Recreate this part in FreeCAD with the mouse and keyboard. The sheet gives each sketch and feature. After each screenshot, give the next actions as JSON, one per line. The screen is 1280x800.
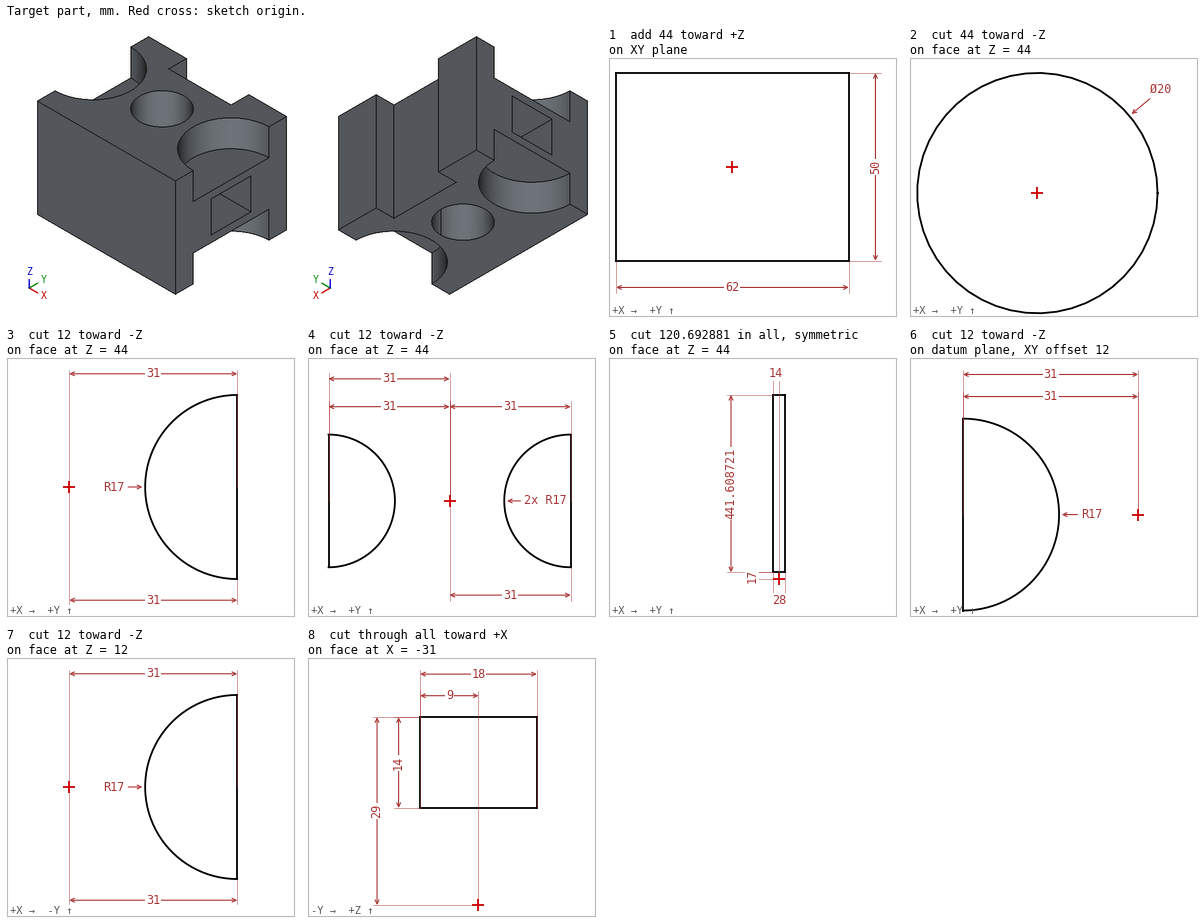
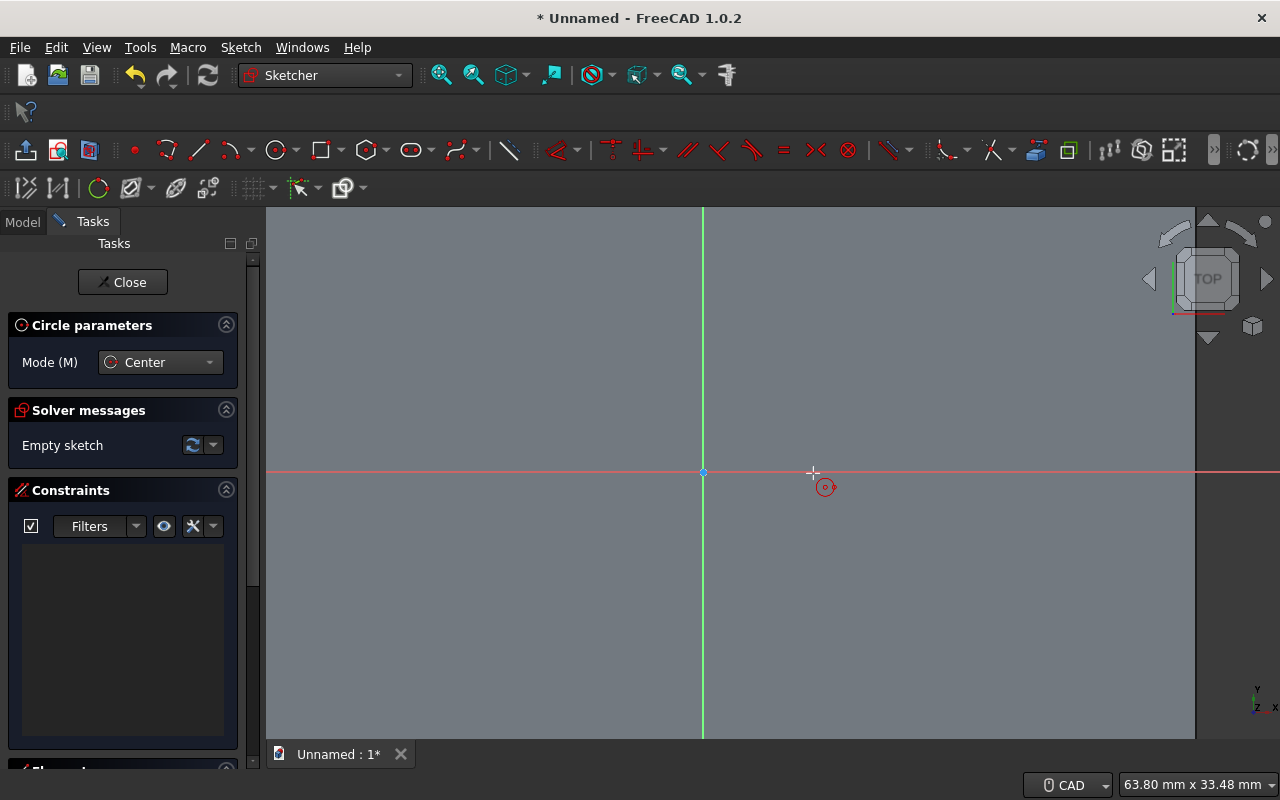
{"action": "left_click", "coordinate": [703, 472]}
{"action": "left_click", "coordinate": [816, 360]}
{"action": "key", "text": "Escape"}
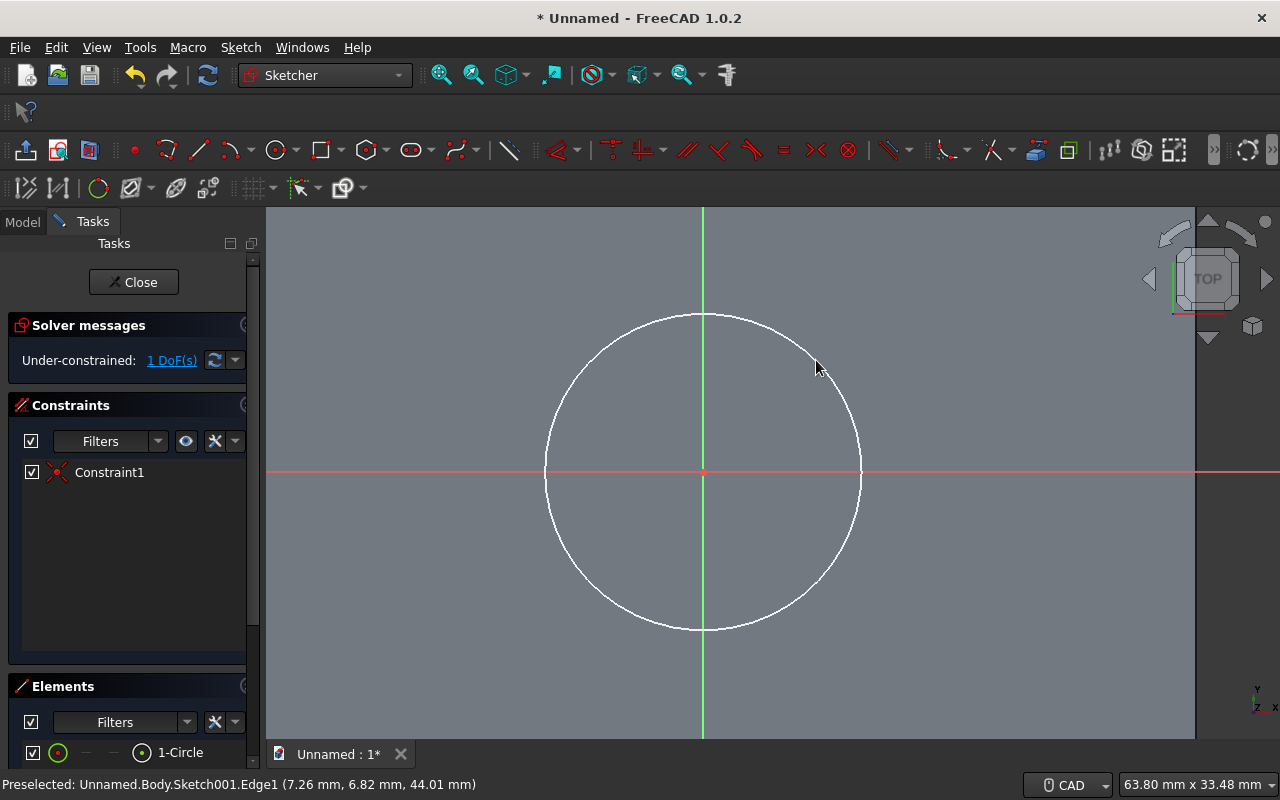
{"action": "key", "text": "d"}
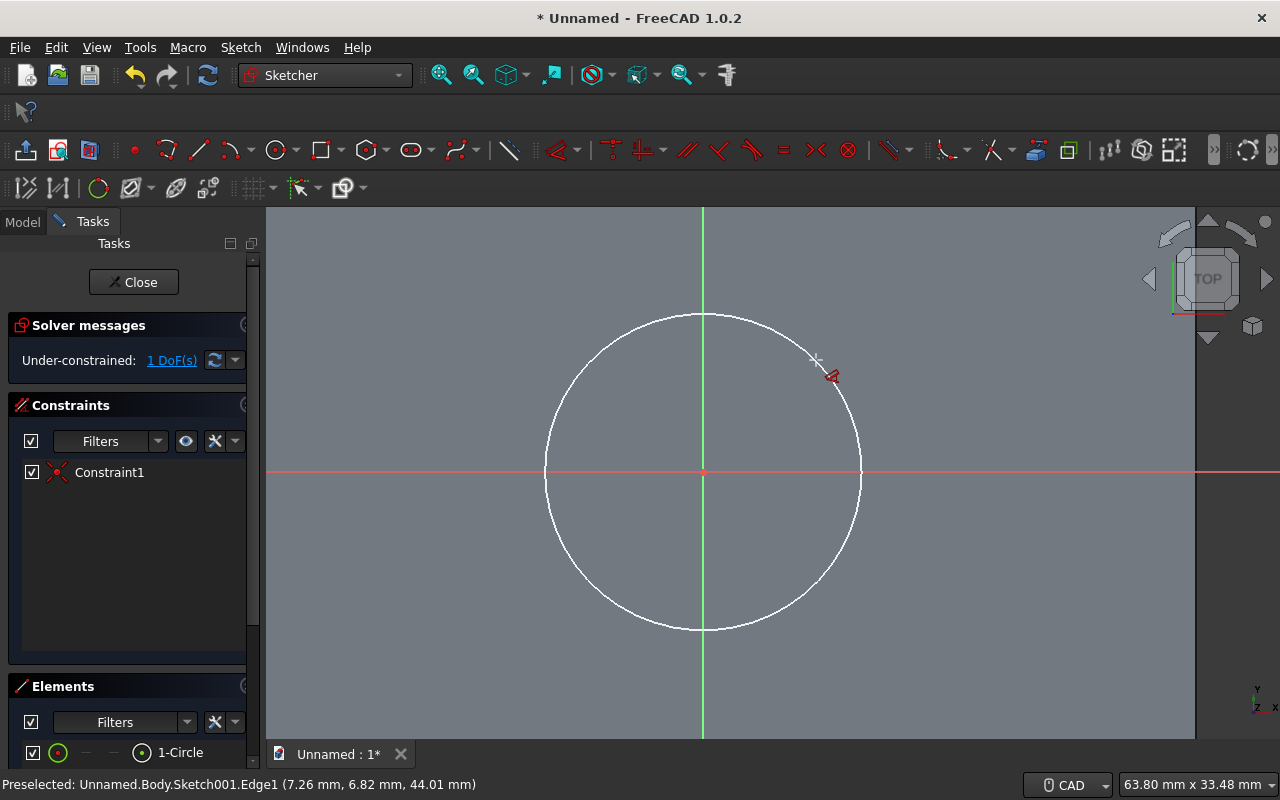
{"action": "left_click", "coordinate": [815, 360]}
{"action": "left_click", "coordinate": [838, 337]}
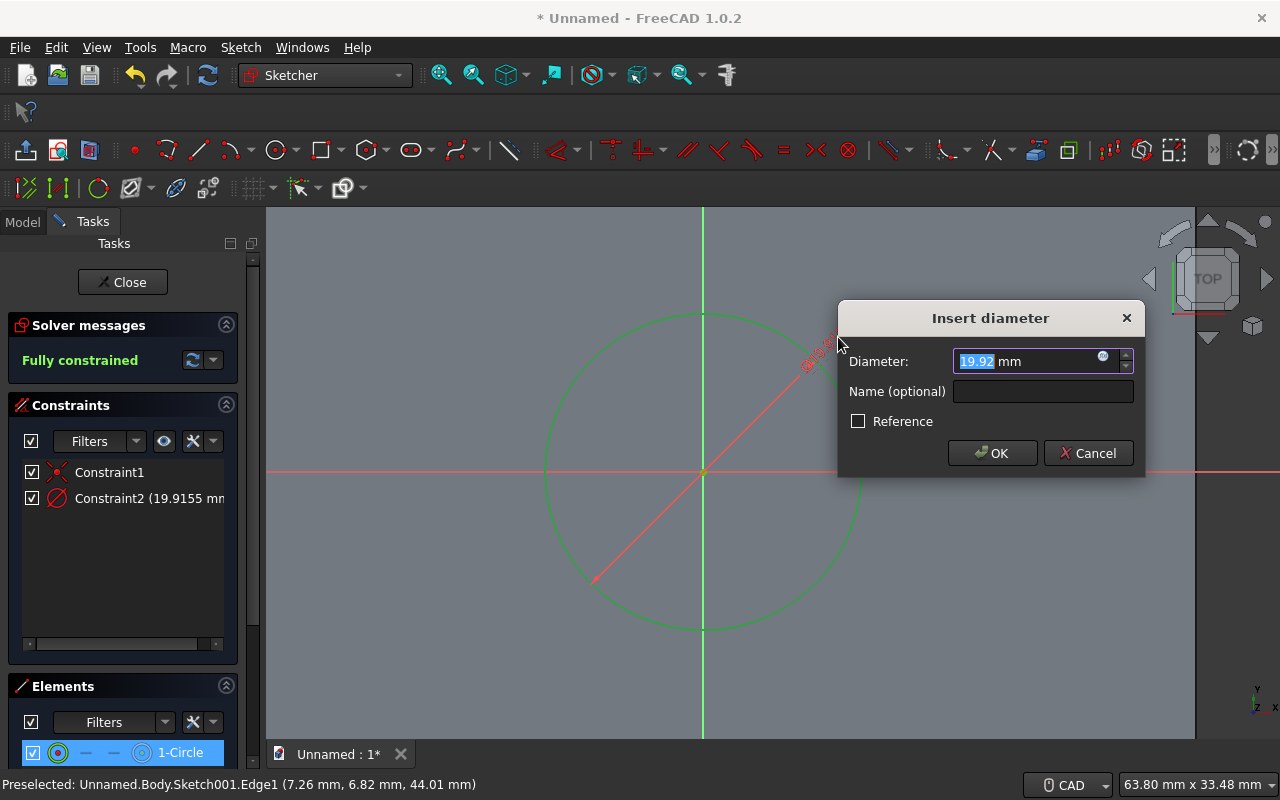
{"action": "type", "text": "20"}
{"action": "key", "text": "Return"}
{"action": "key", "text": "Escape"}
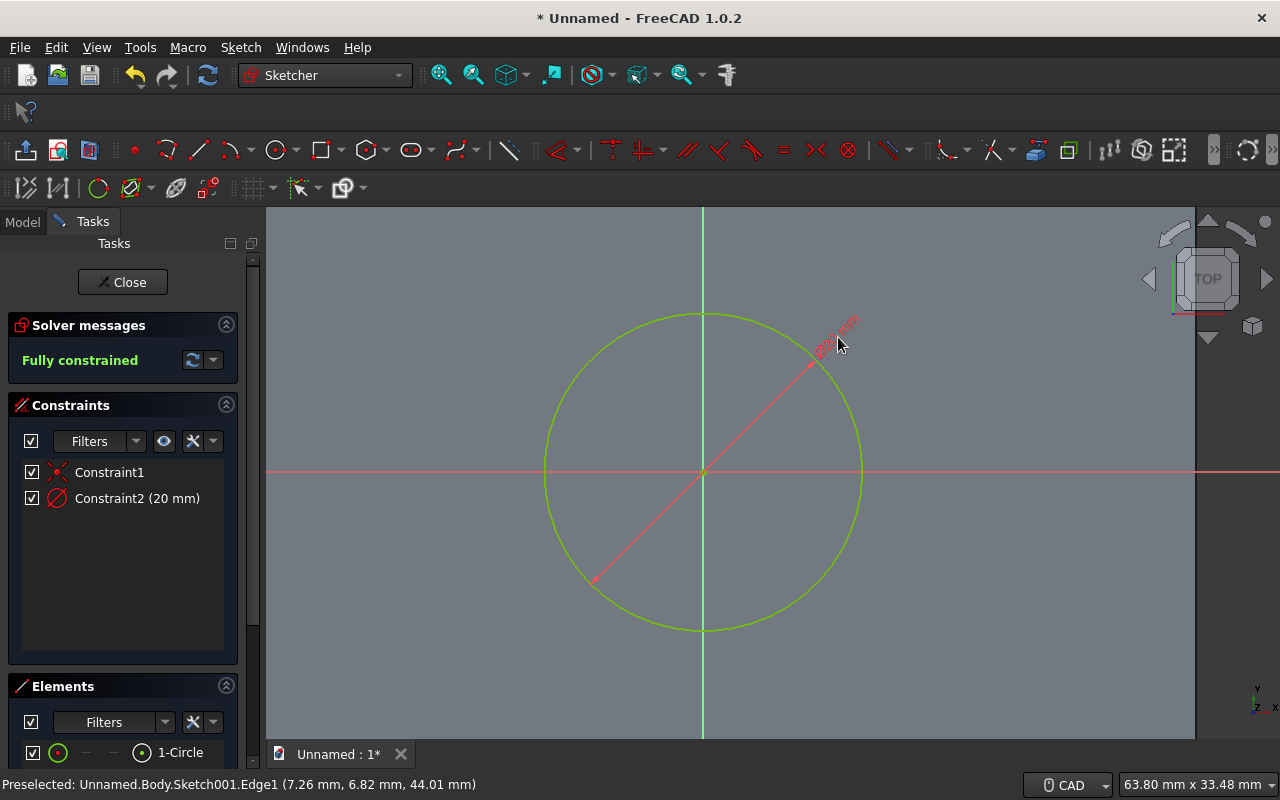
{"action": "left_click", "coordinate": [123, 282]}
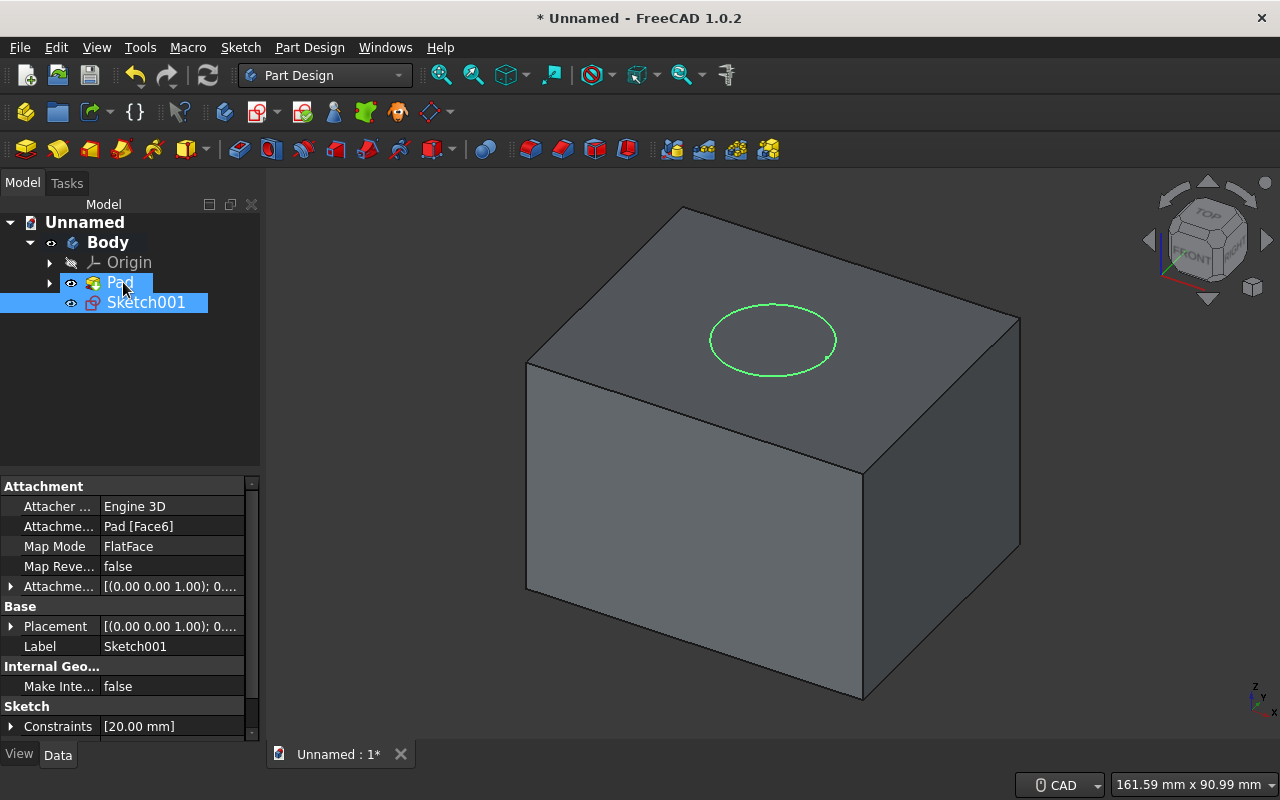
{"action": "left_click", "coordinate": [240, 150]}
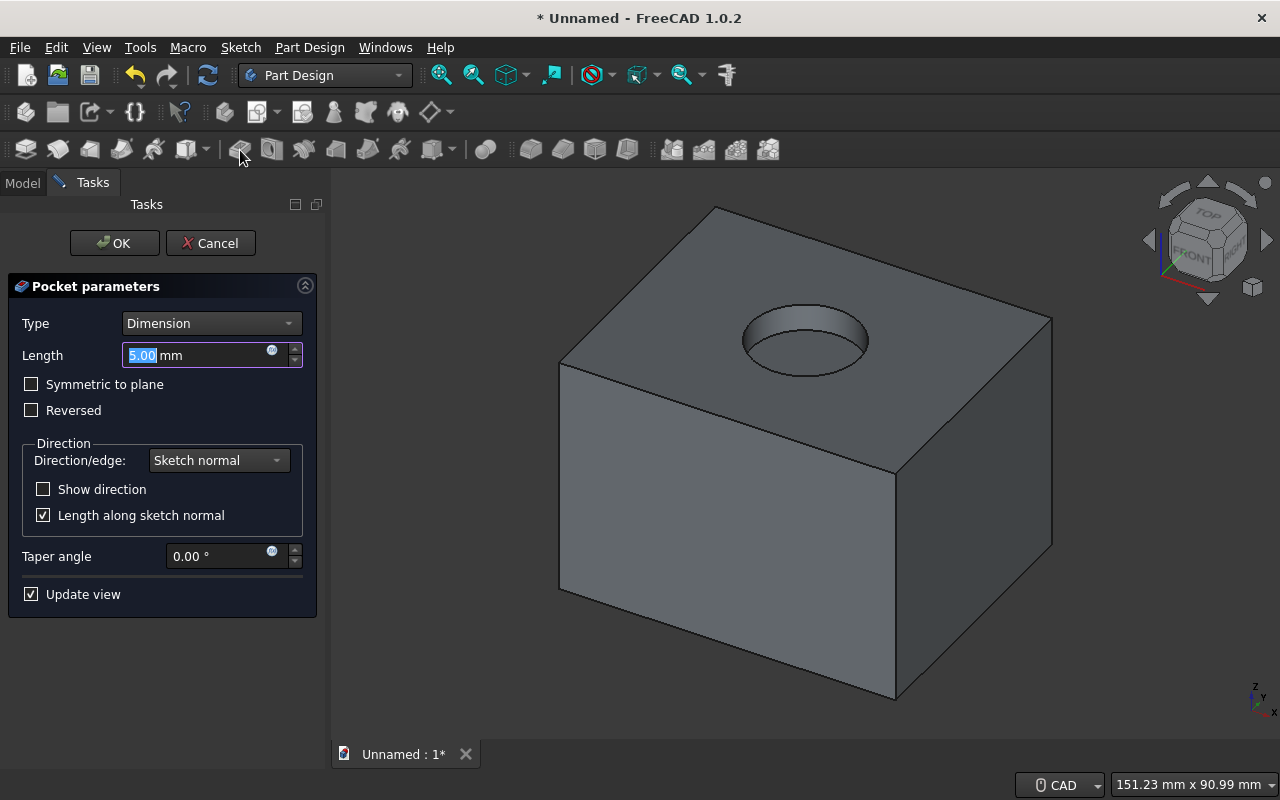
{"action": "type", "text": "44"}
{"action": "key", "text": "Tab"}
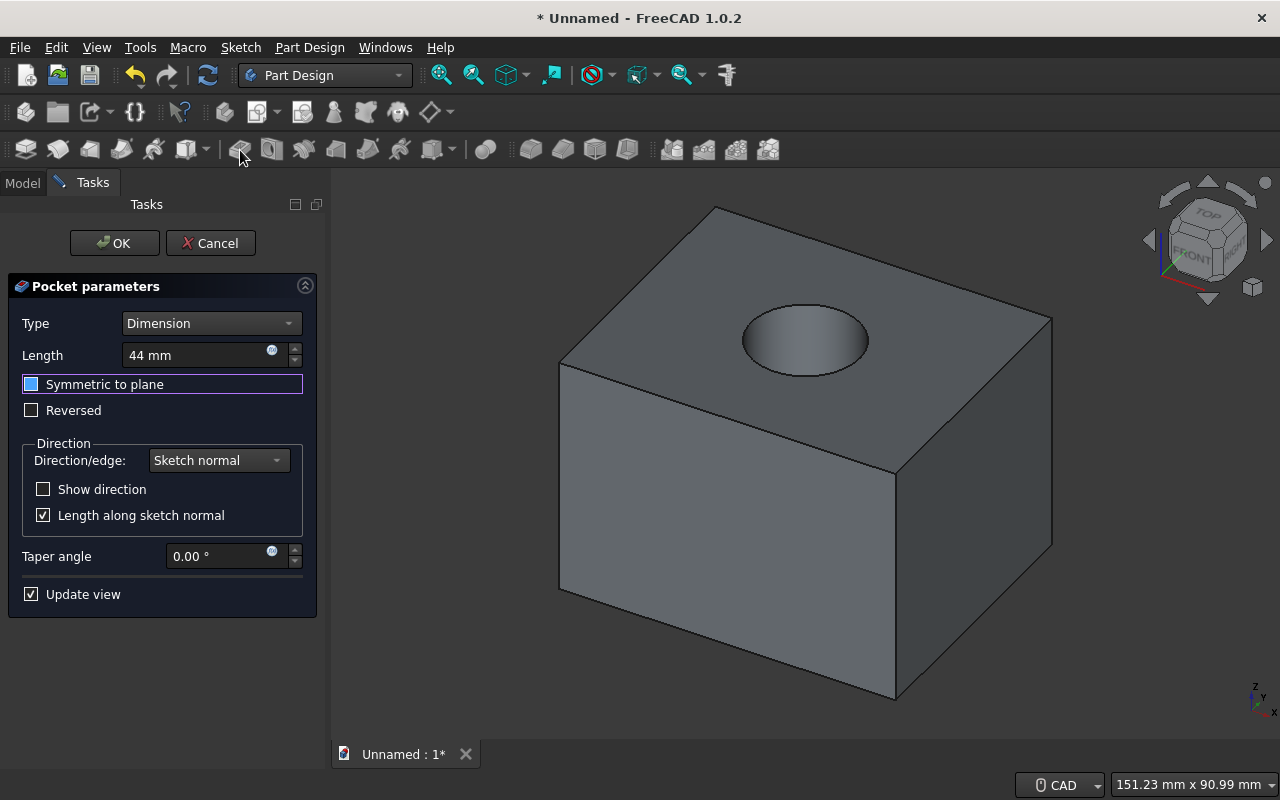
{"action": "left_click", "coordinate": [115, 243]}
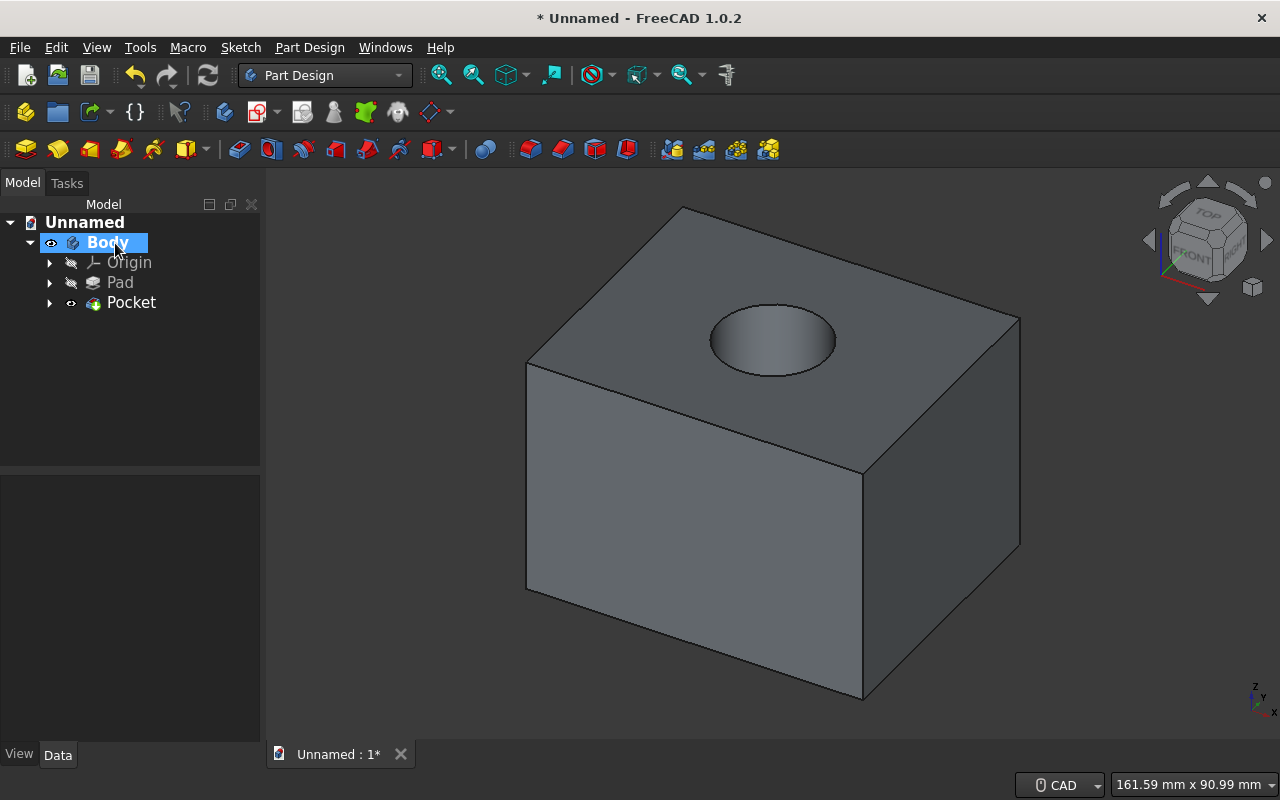
{"action": "left_click", "coordinate": [914, 327]}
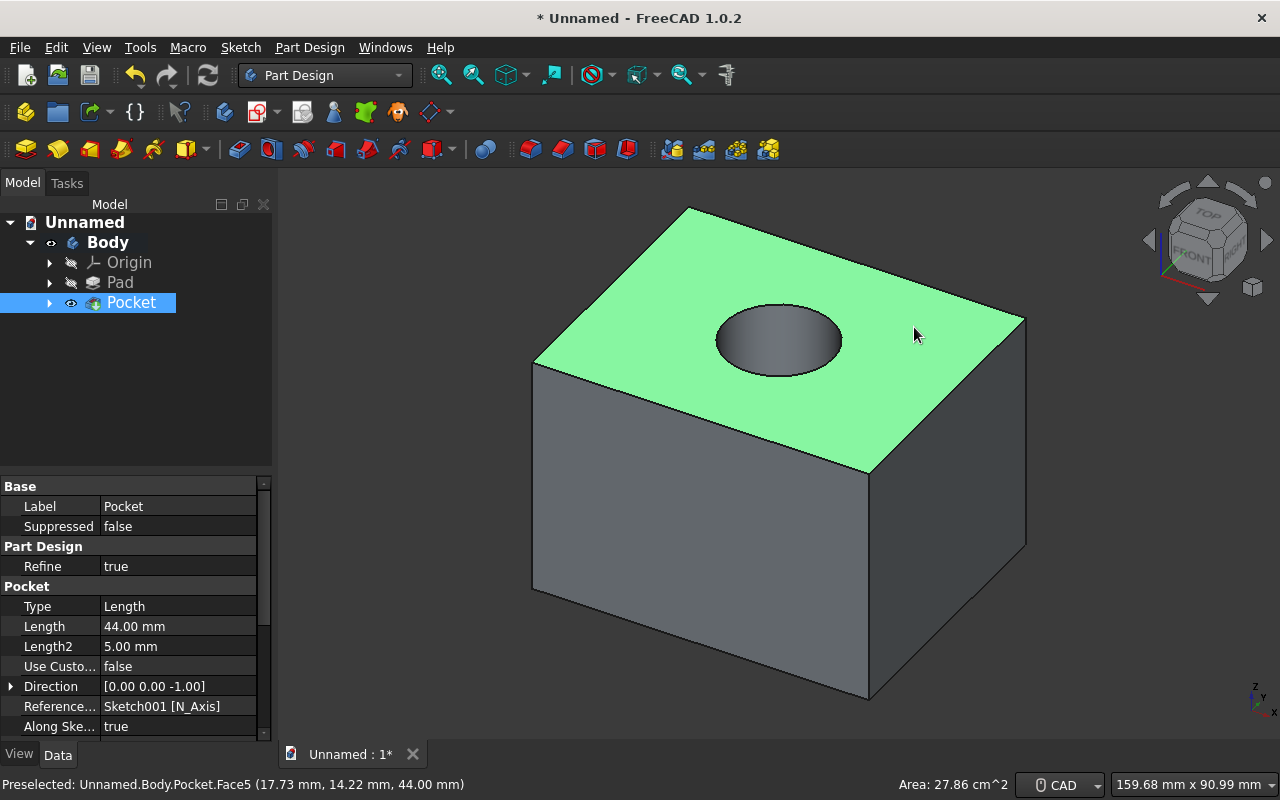
{"action": "left_click", "coordinate": [258, 112]}